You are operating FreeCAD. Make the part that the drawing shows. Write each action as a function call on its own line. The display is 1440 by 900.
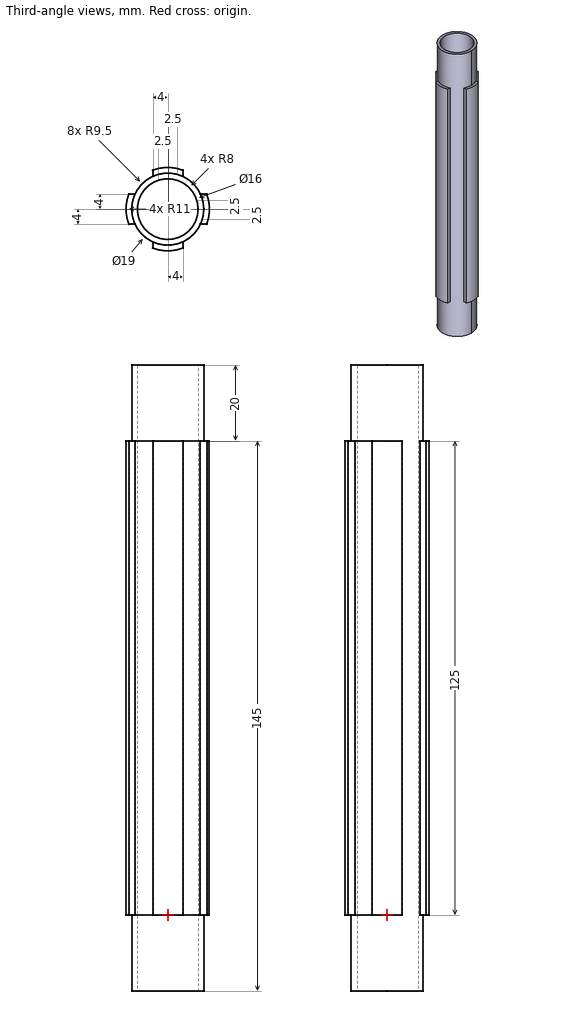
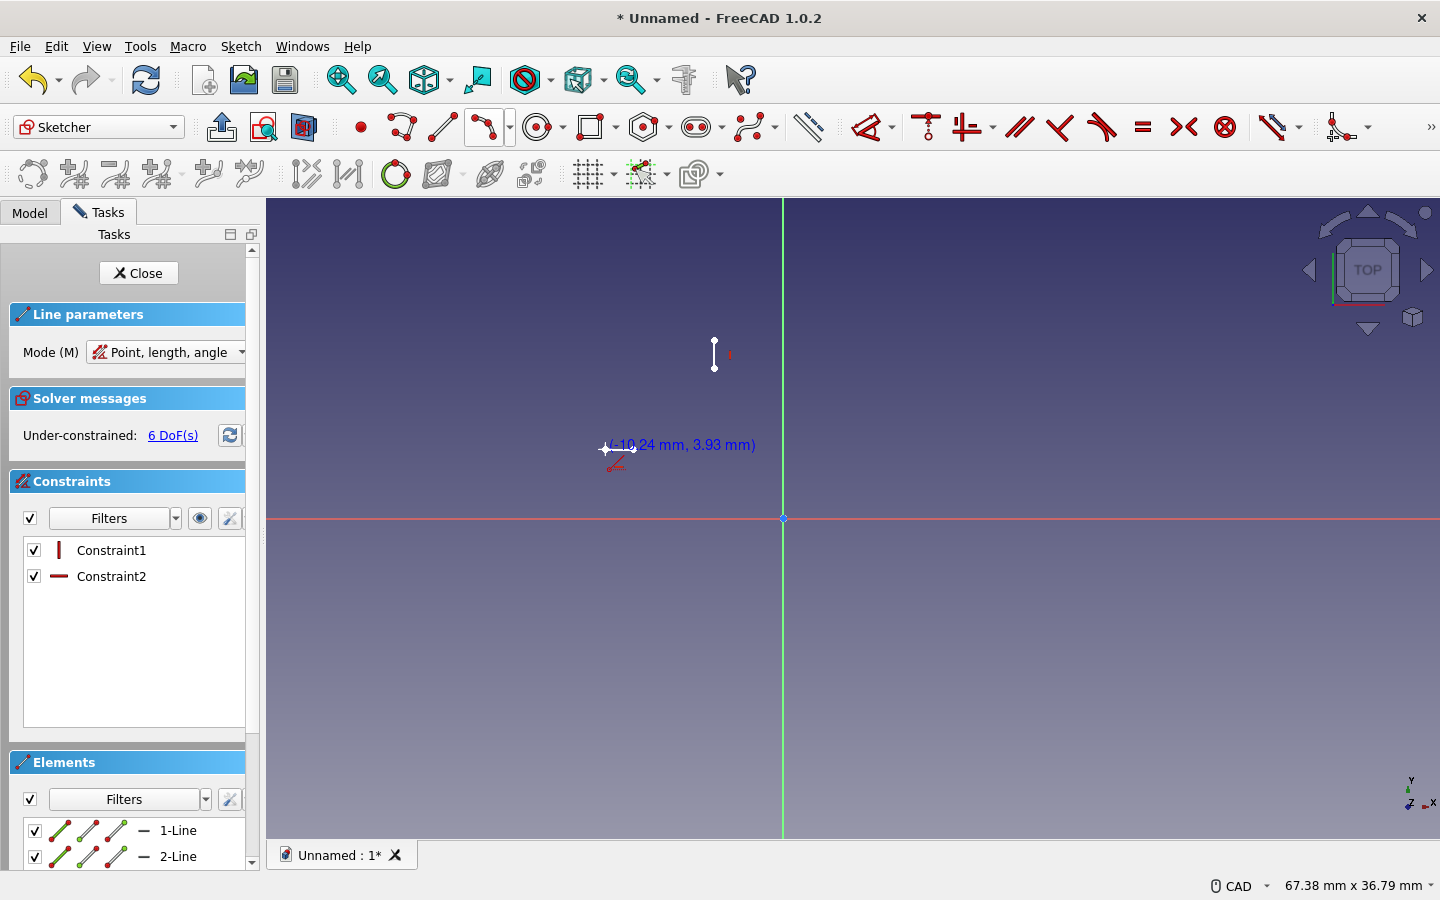
click(605, 588)
click(633, 588)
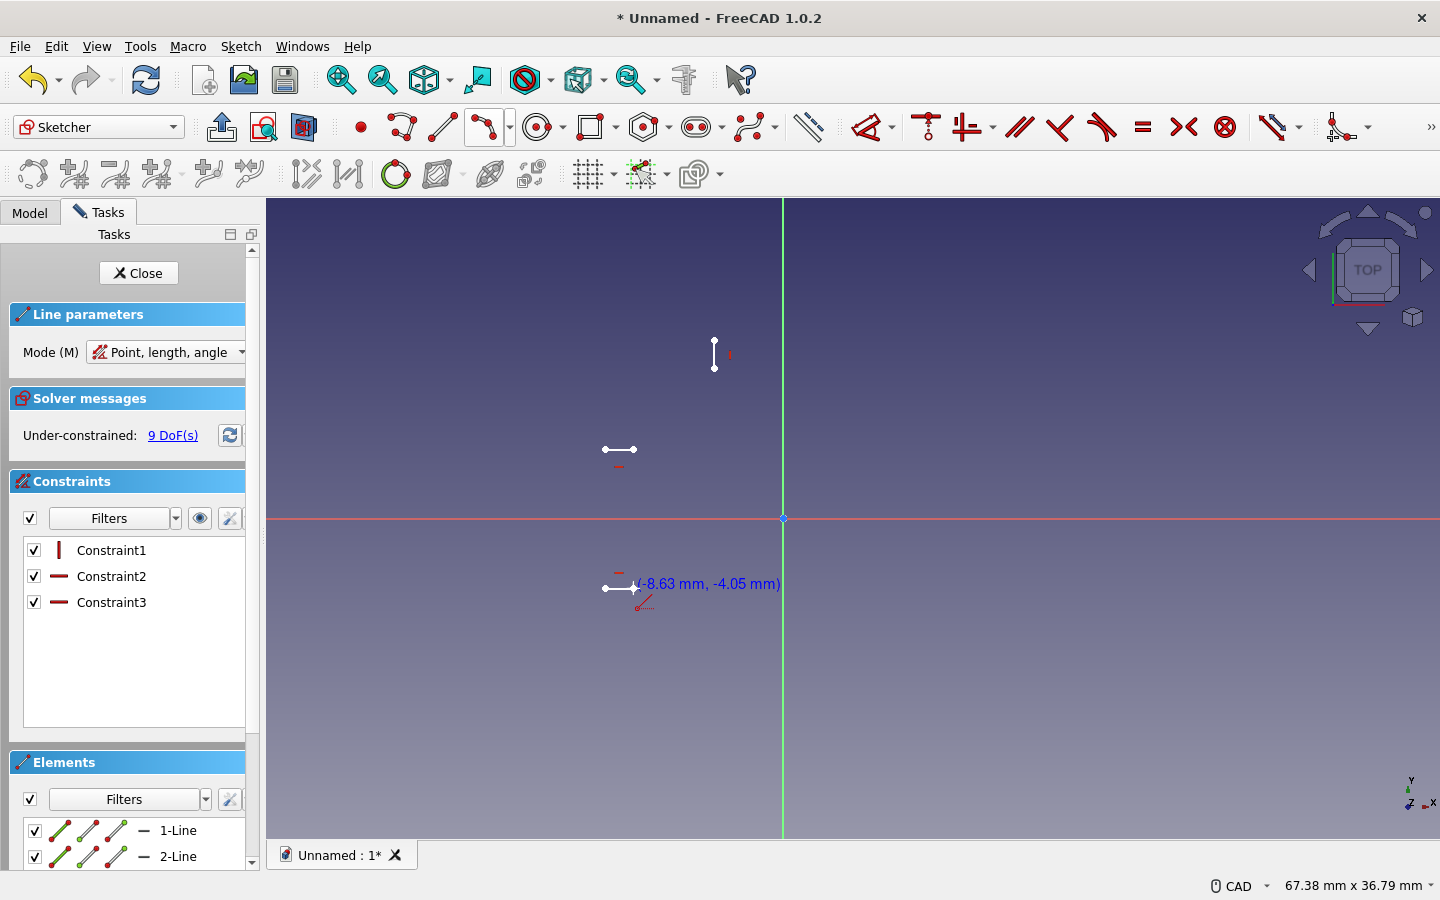
click(714, 669)
click(714, 697)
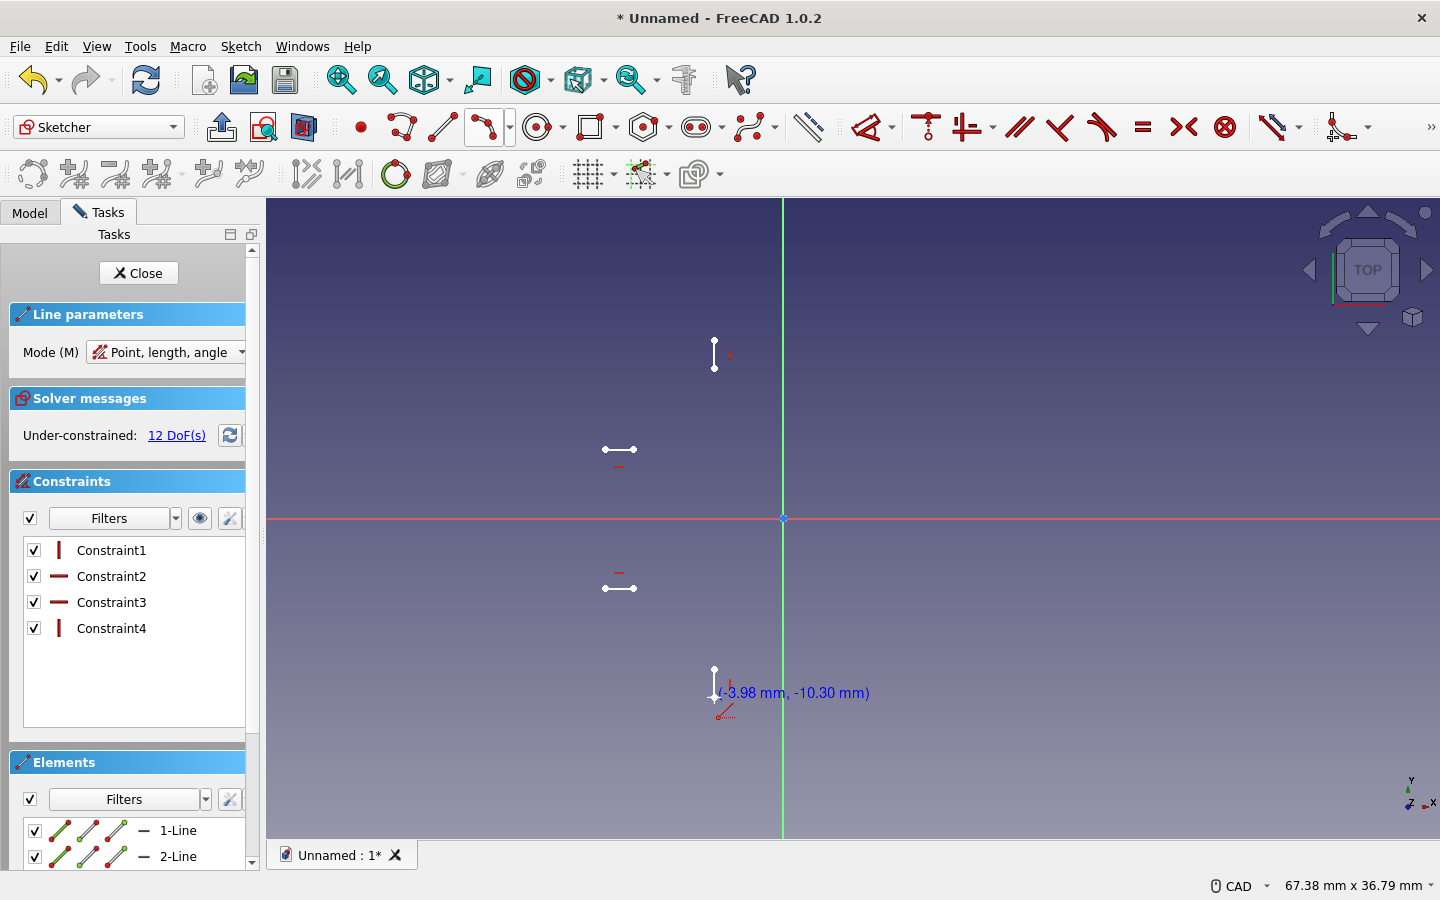
click(853, 697)
click(853, 669)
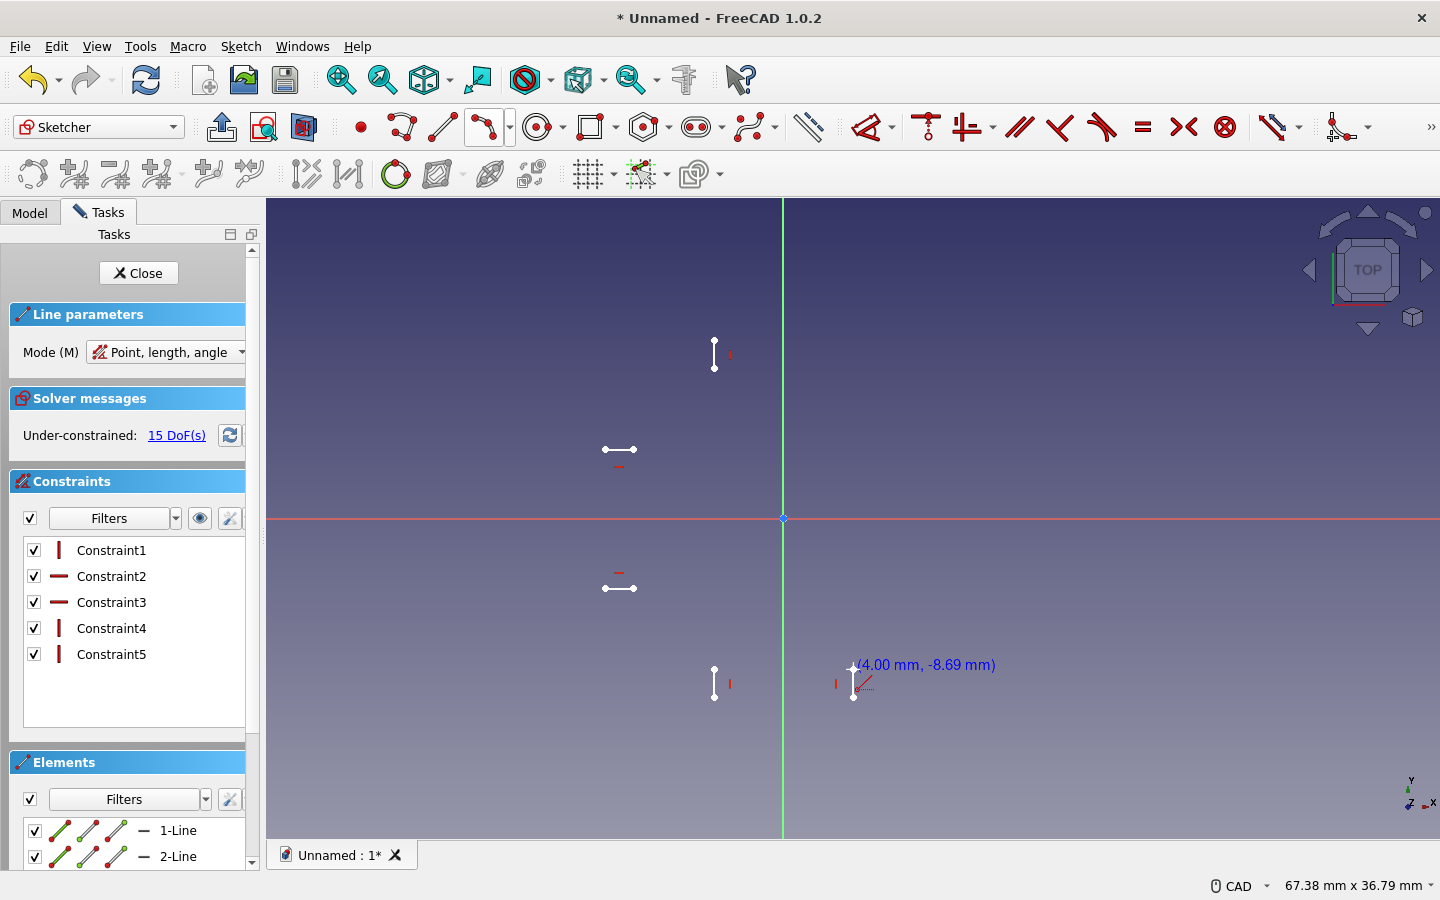
click(933, 588)
click(962, 588)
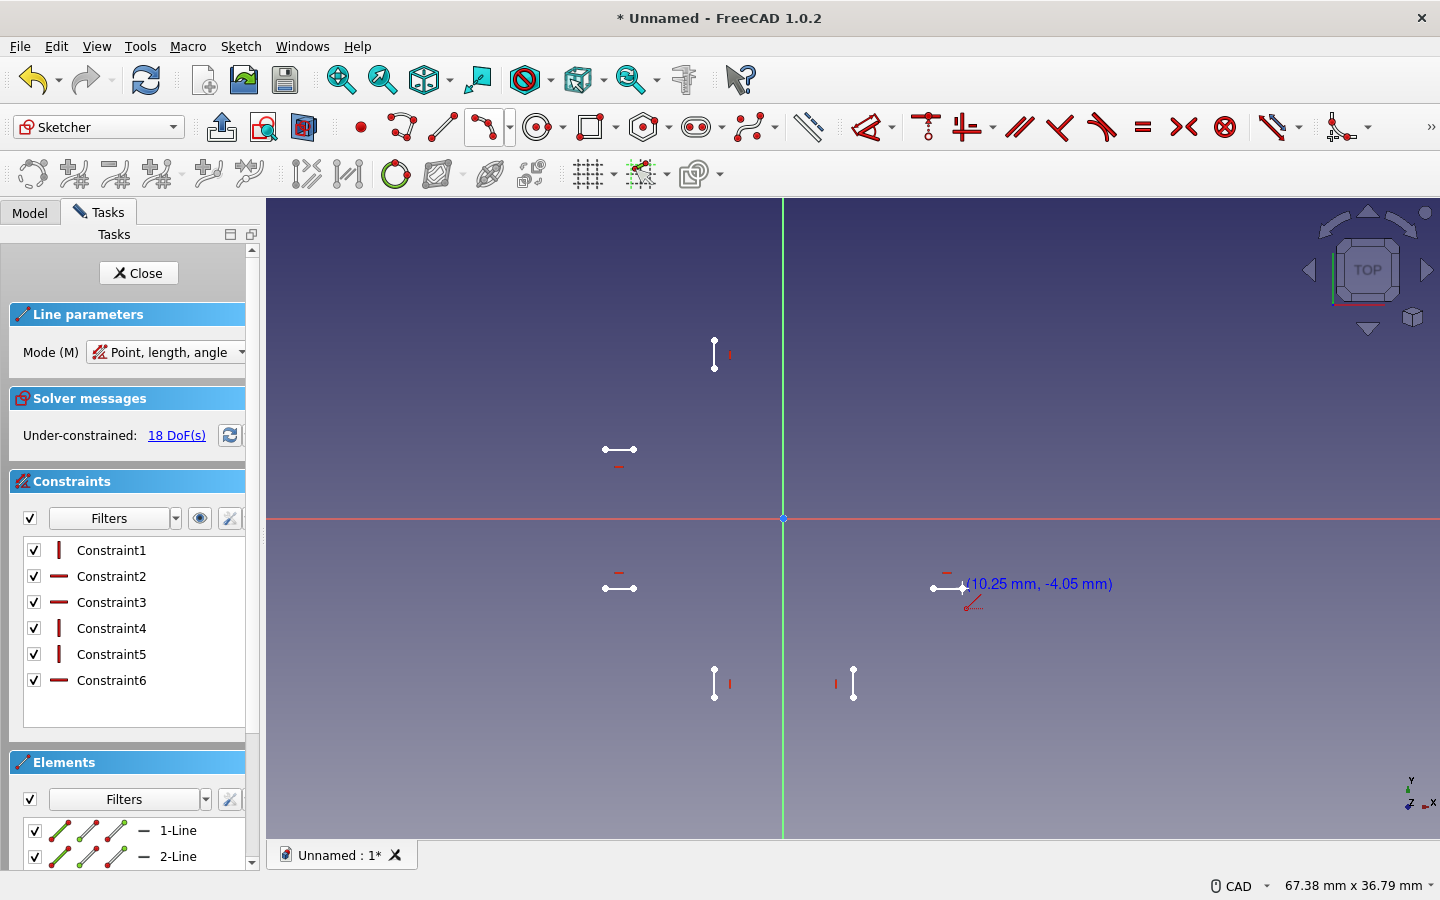
click(962, 449)
click(933, 449)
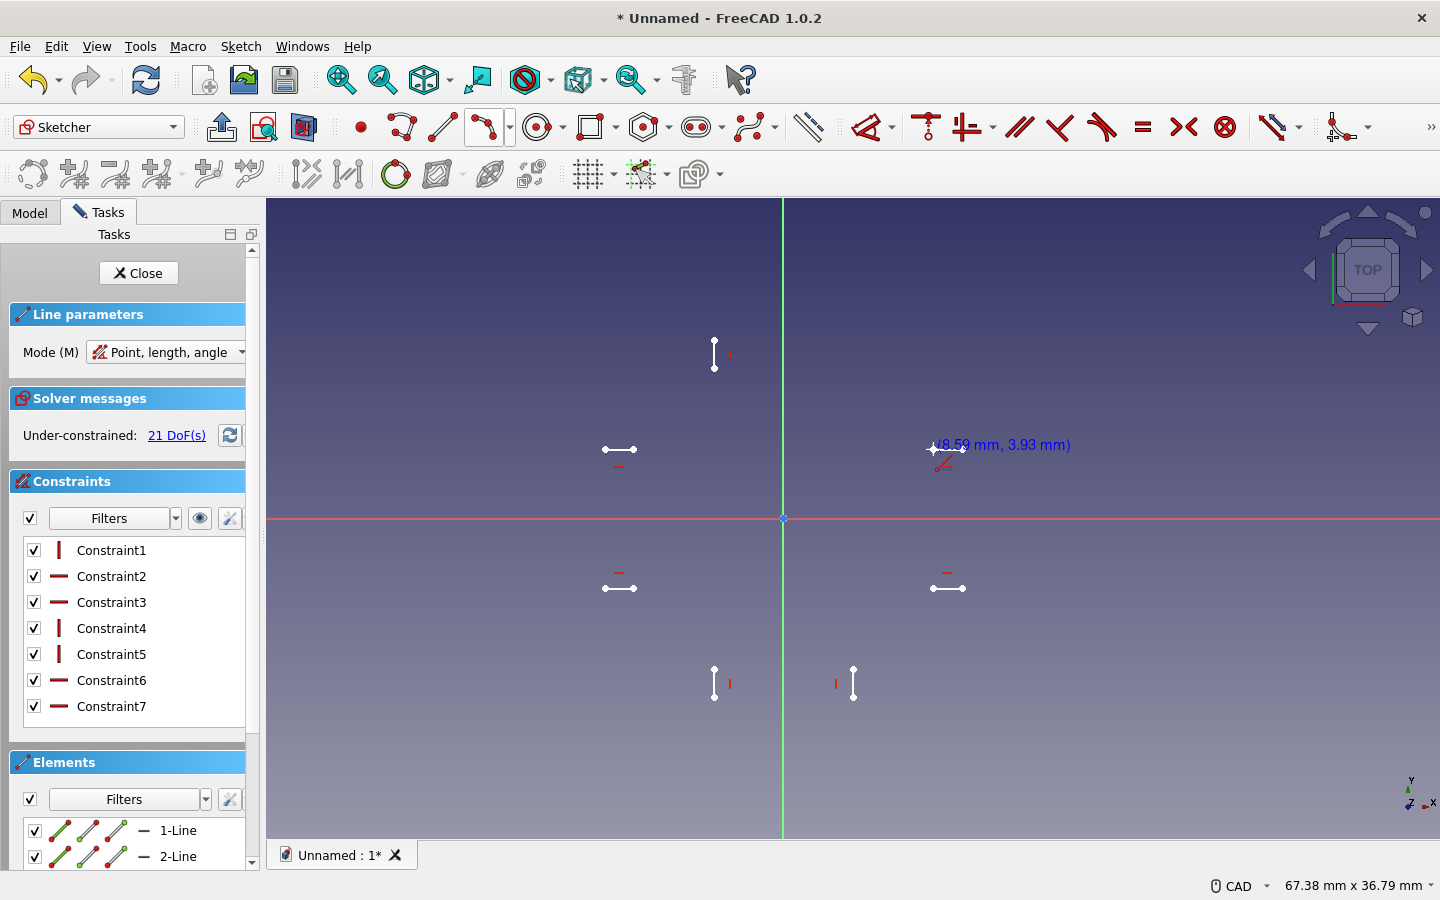
click(853, 368)
click(853, 340)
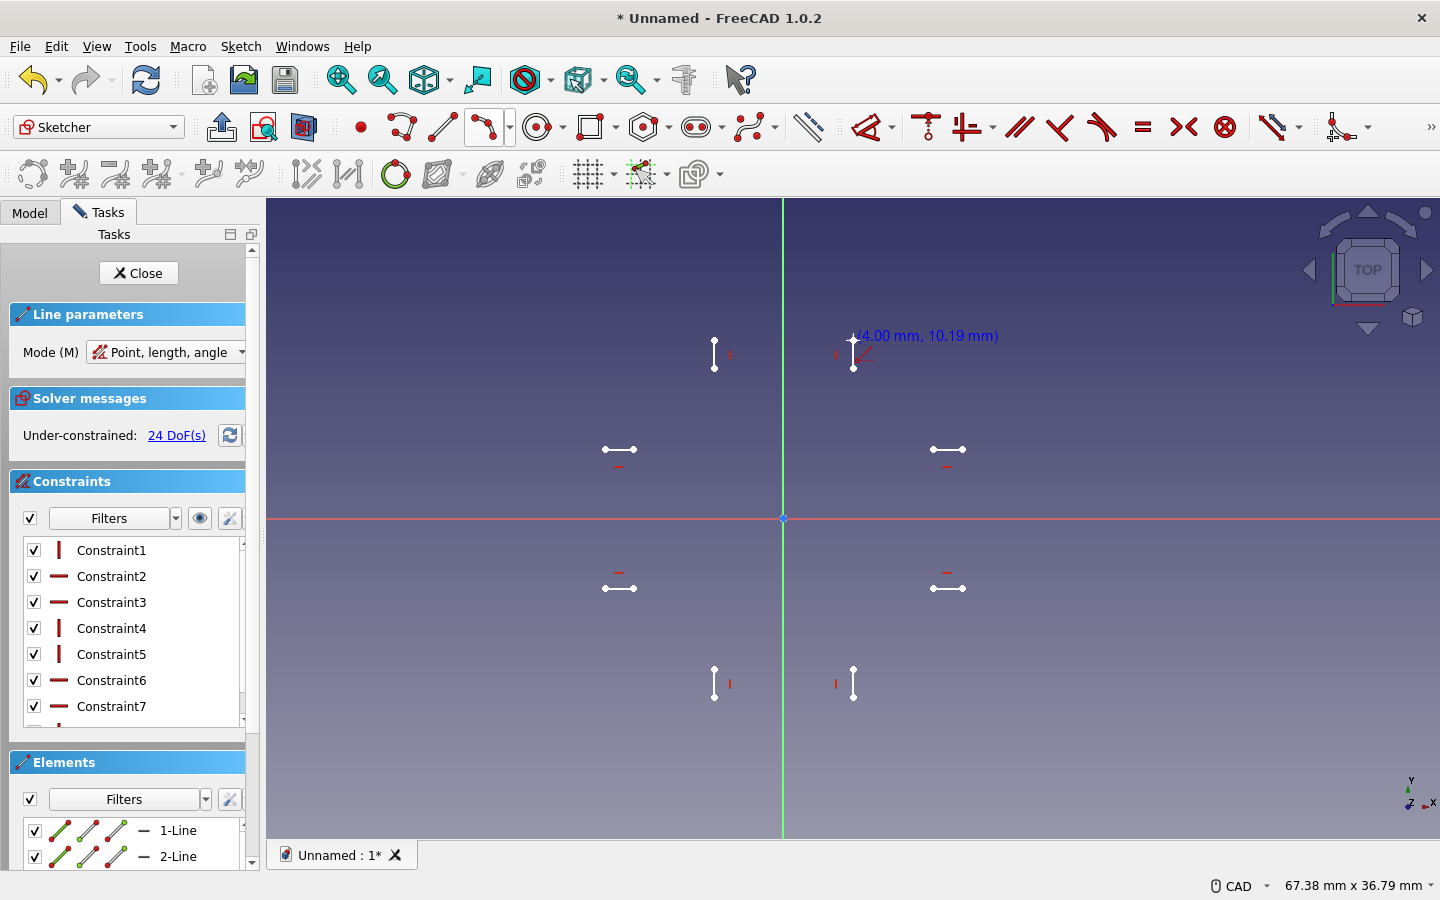
click(484, 128)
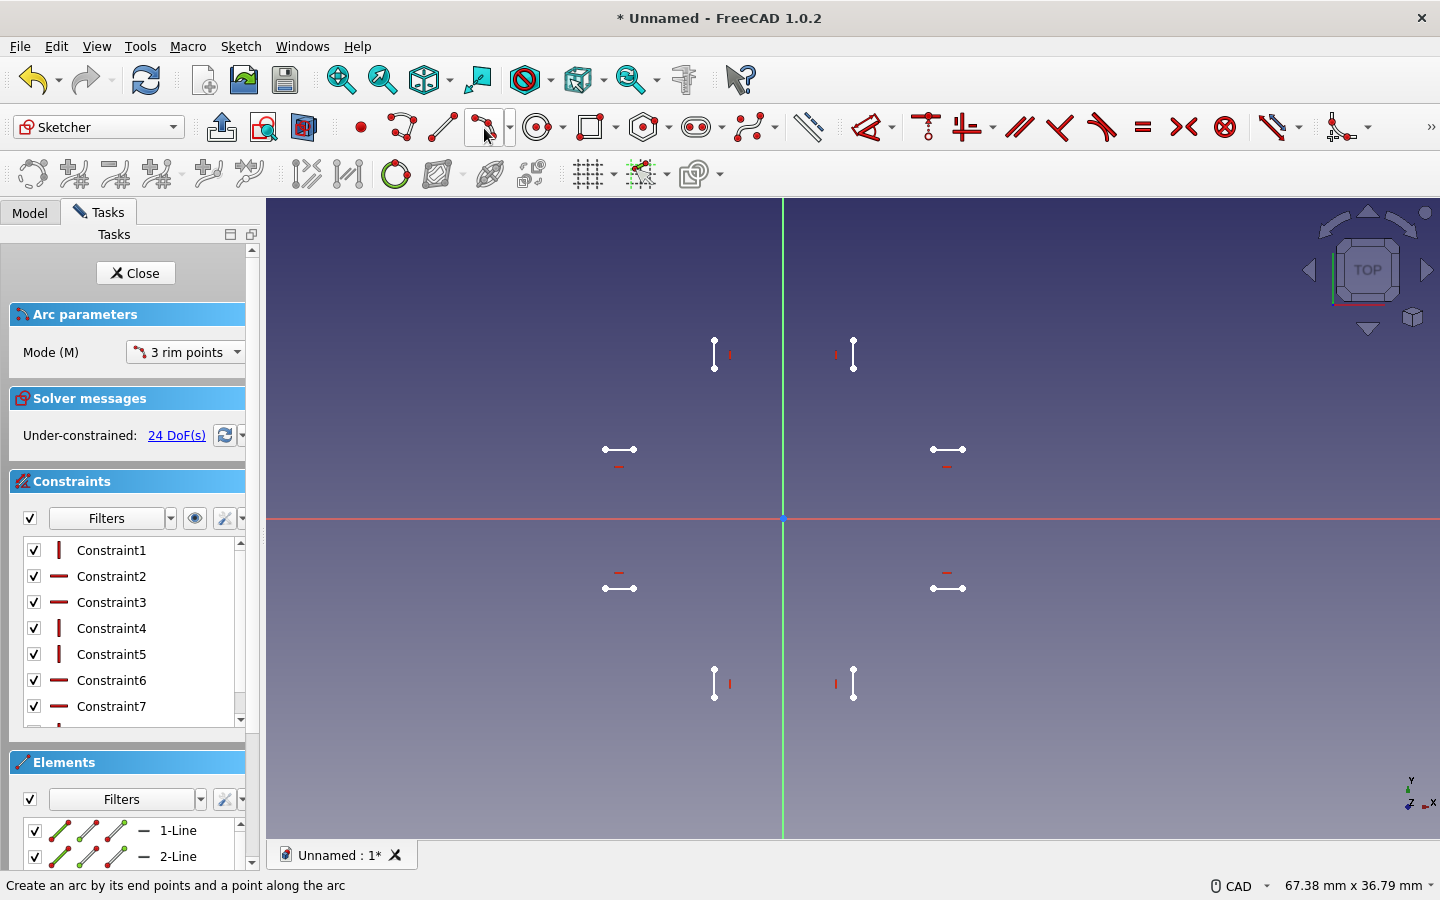
click(714, 369)
click(633, 450)